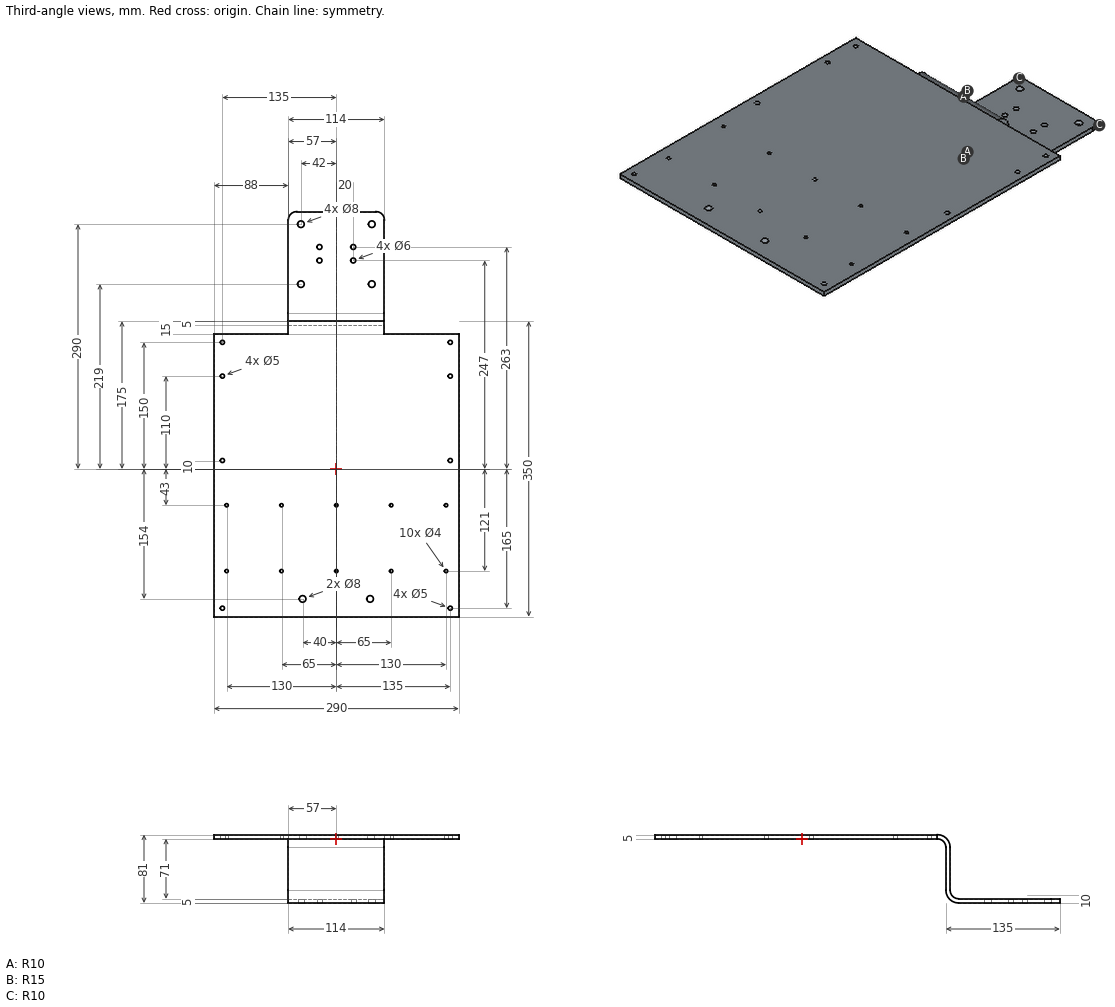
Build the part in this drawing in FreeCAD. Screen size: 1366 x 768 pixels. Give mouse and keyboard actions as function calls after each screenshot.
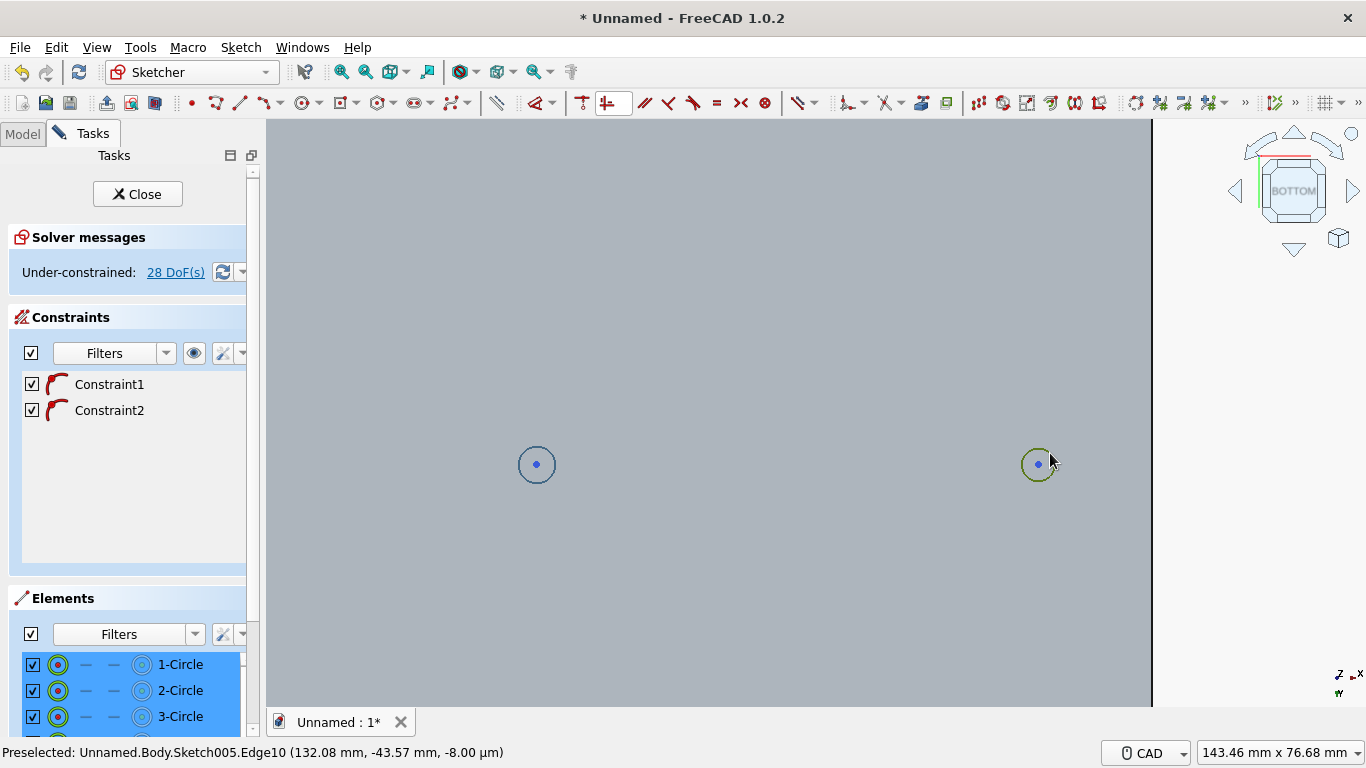
click(718, 104)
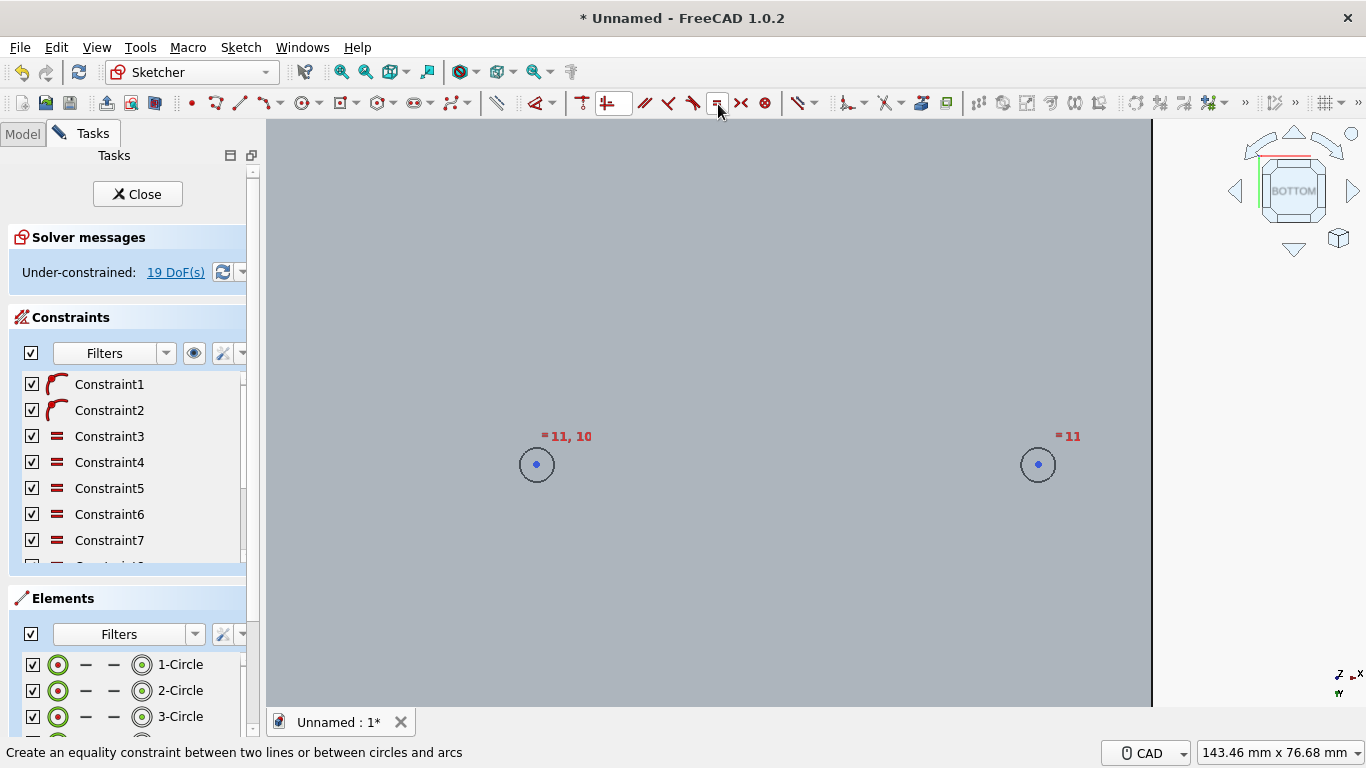
scroll(1052, 453, down, 6)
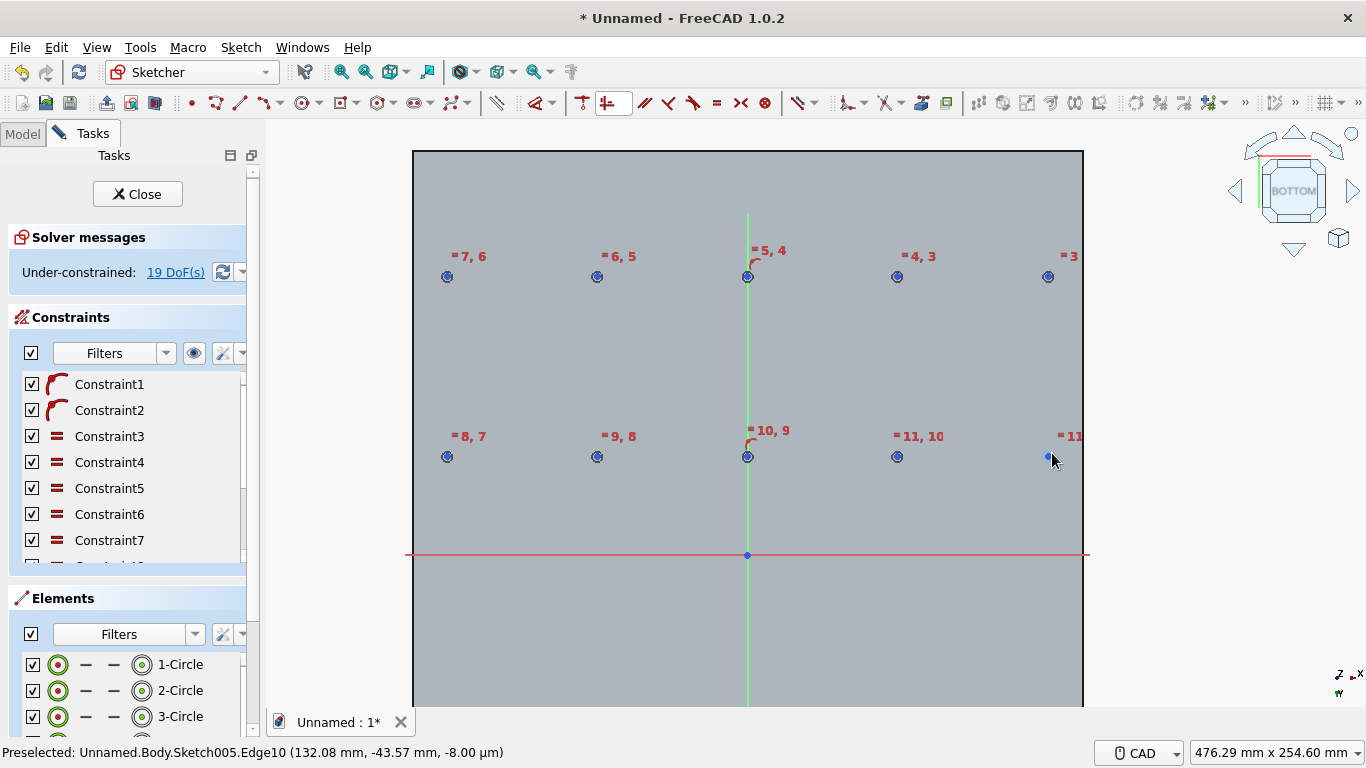
click(897, 277)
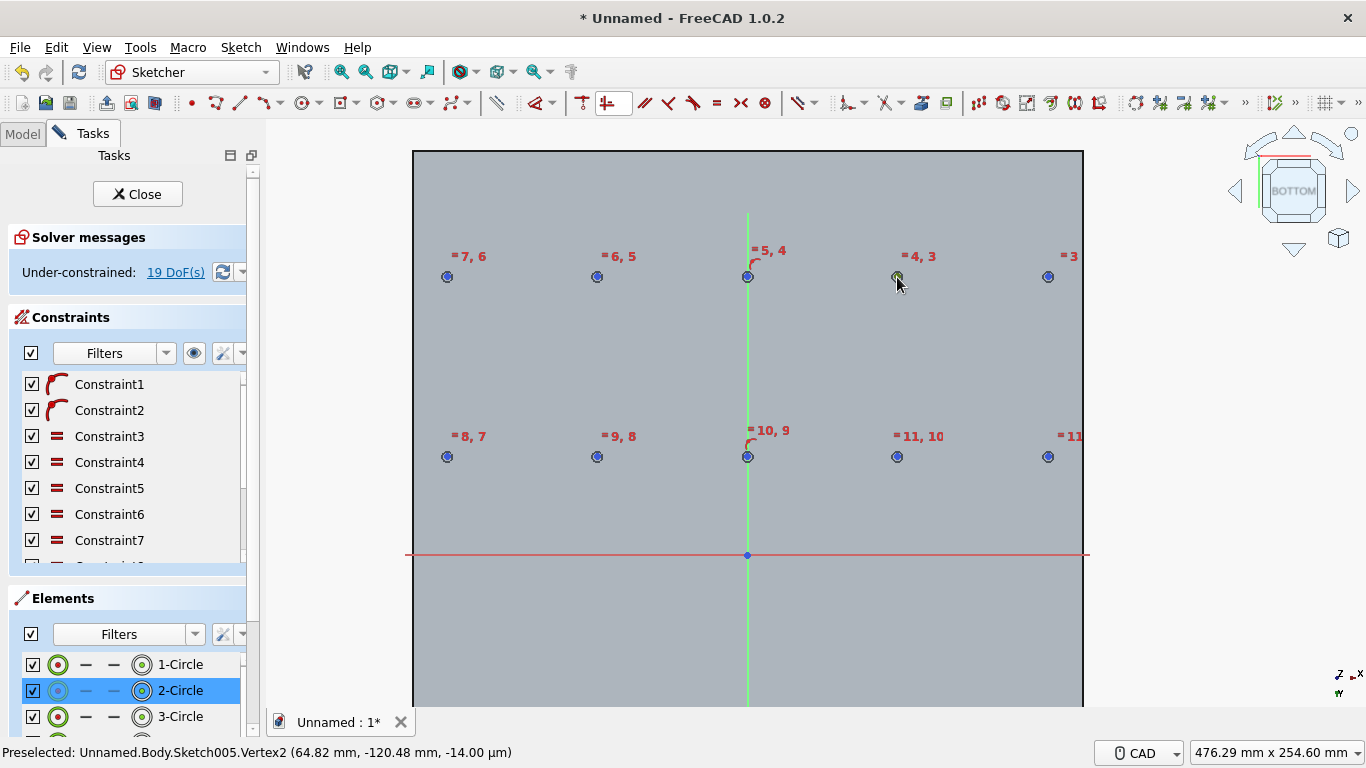
click(597, 277)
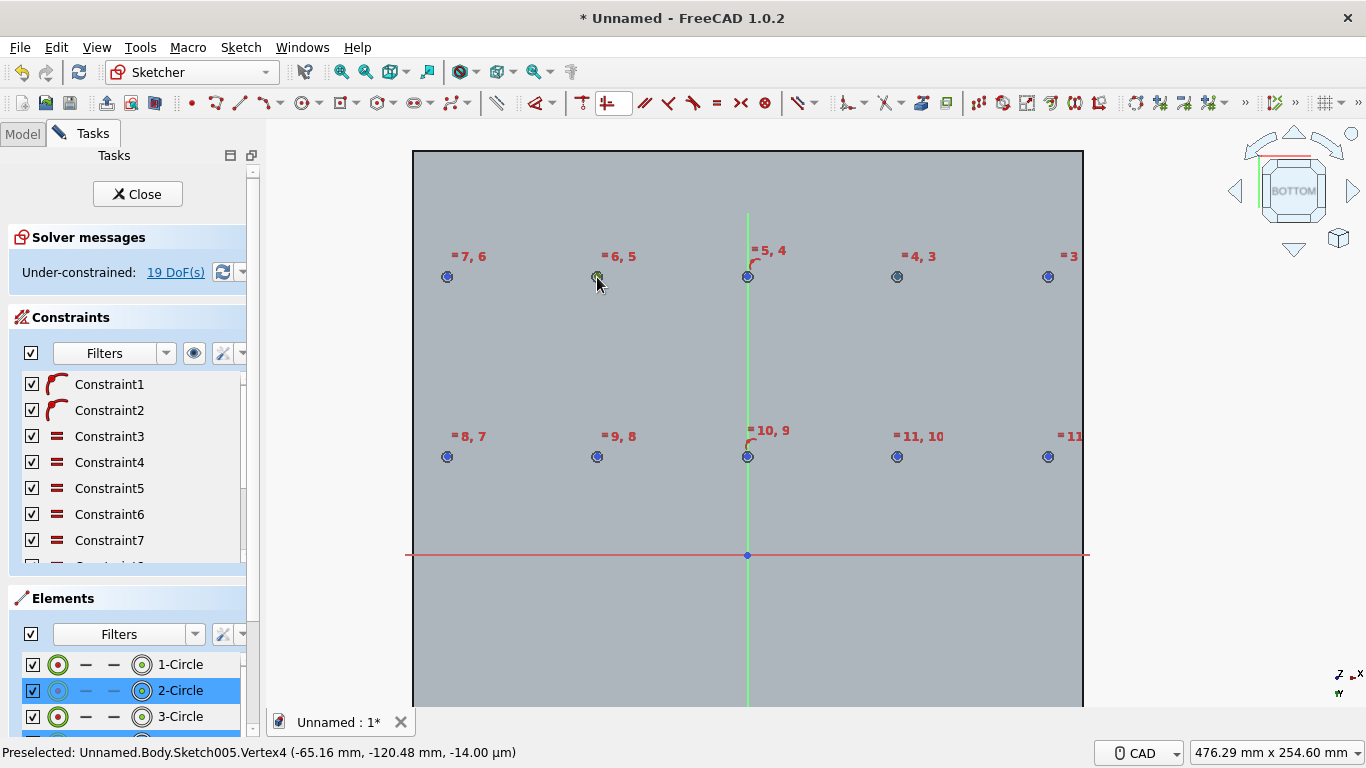
click(748, 641)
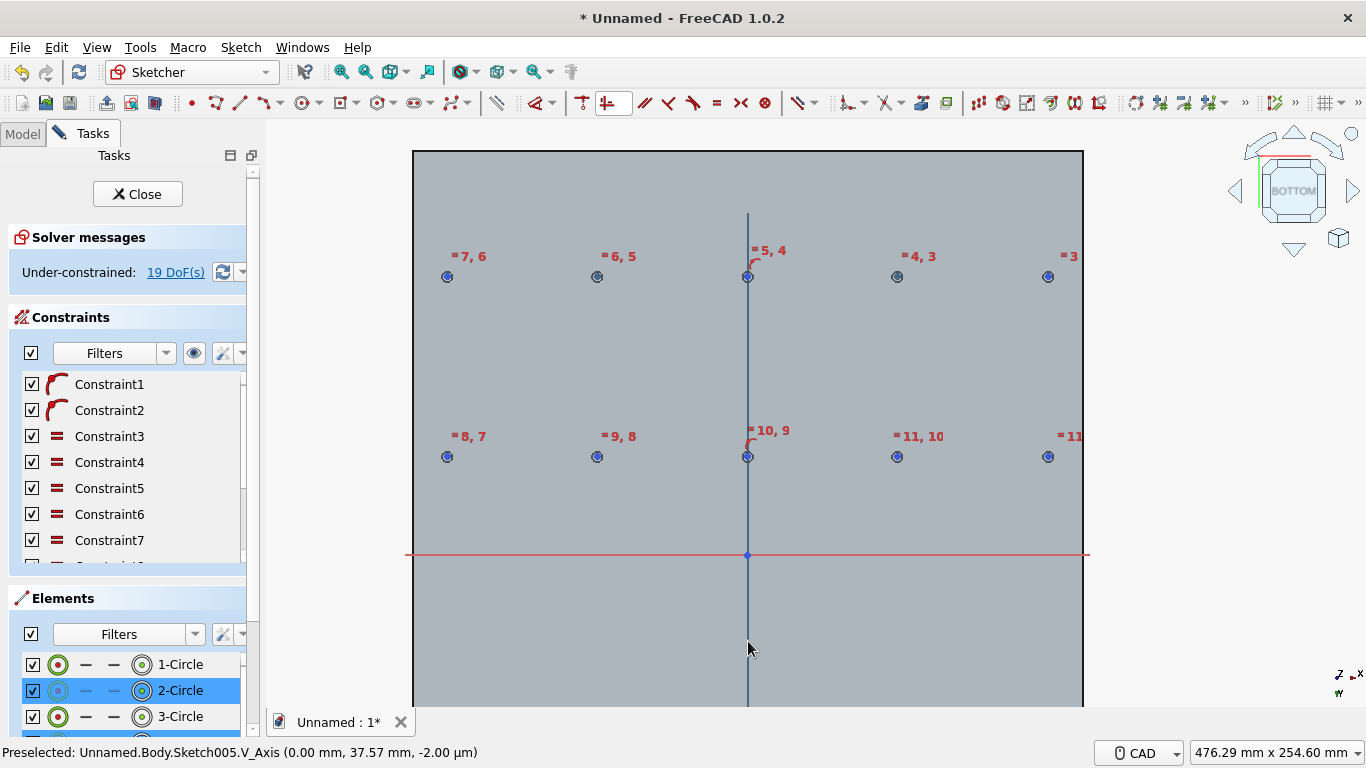
key(s)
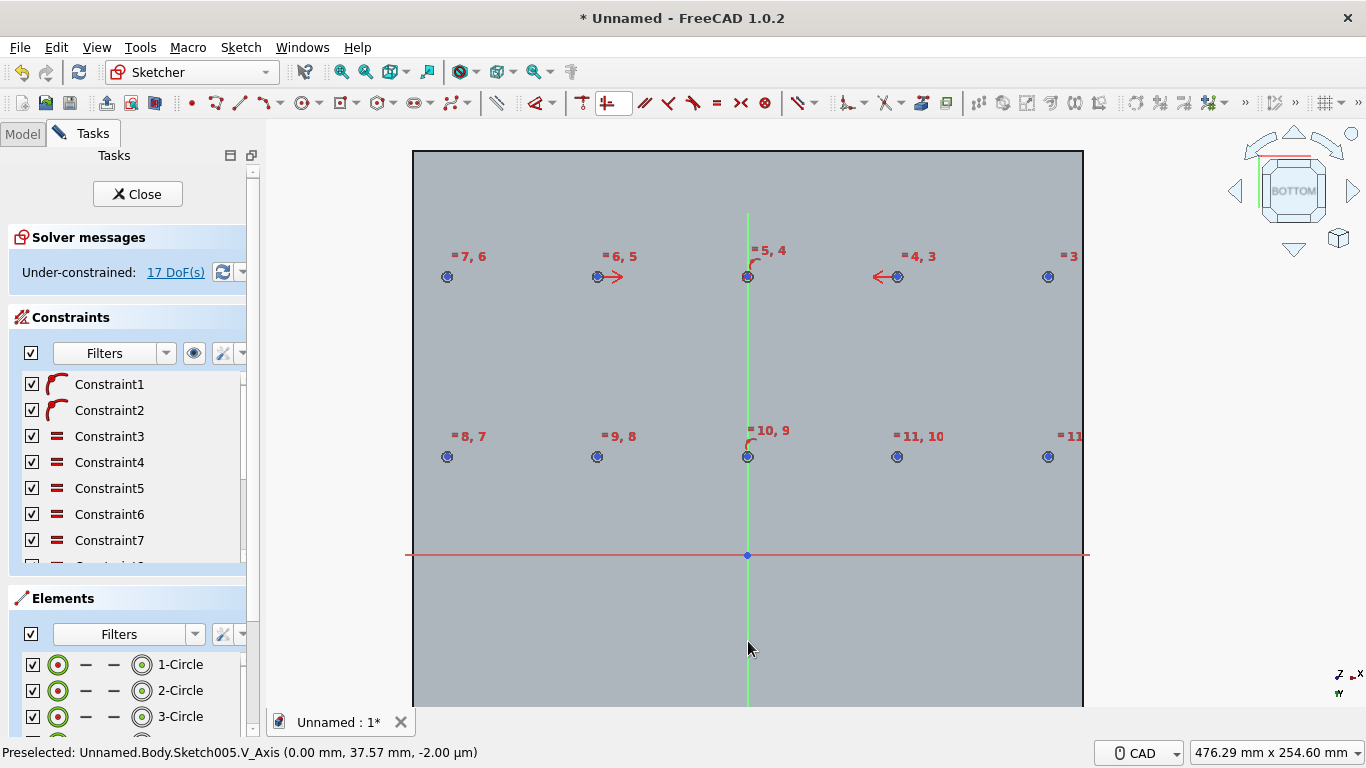
click(1048, 277)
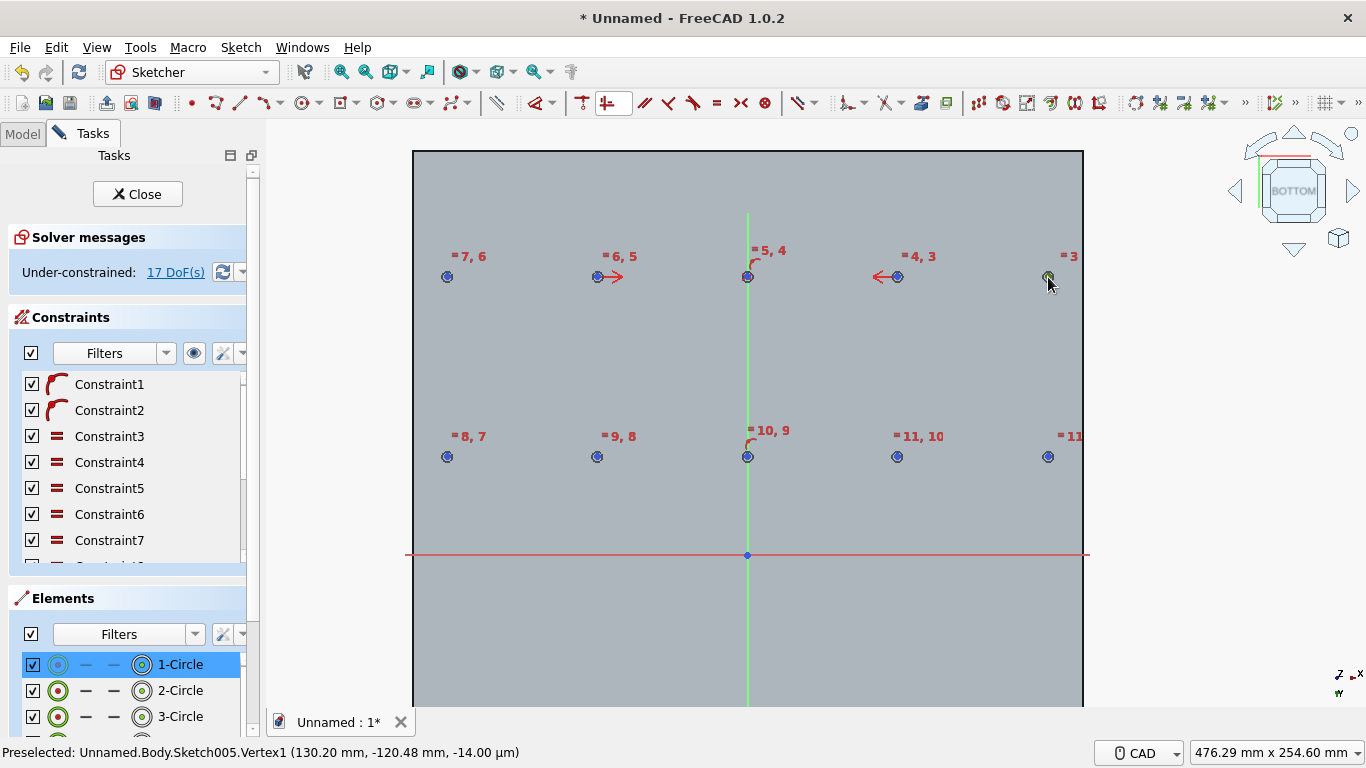
click(447, 277)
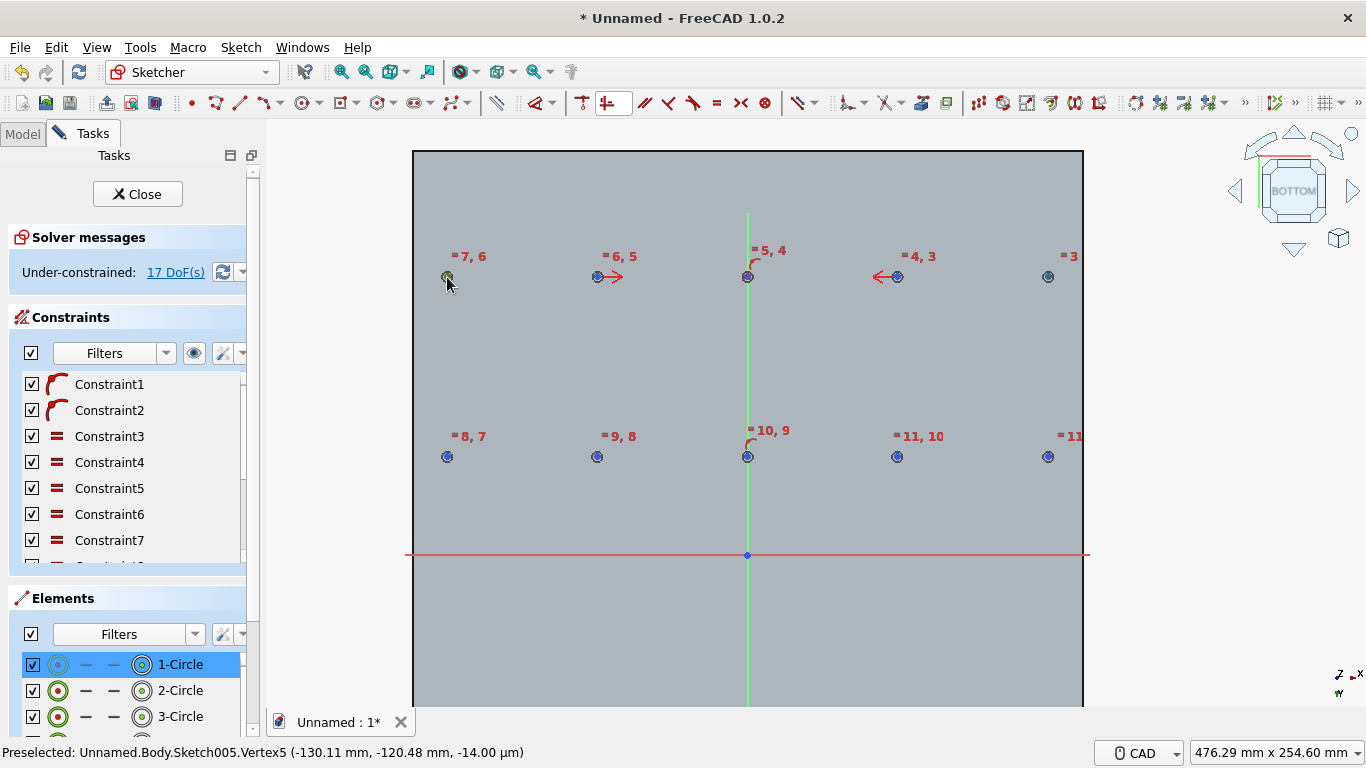
click(748, 641)